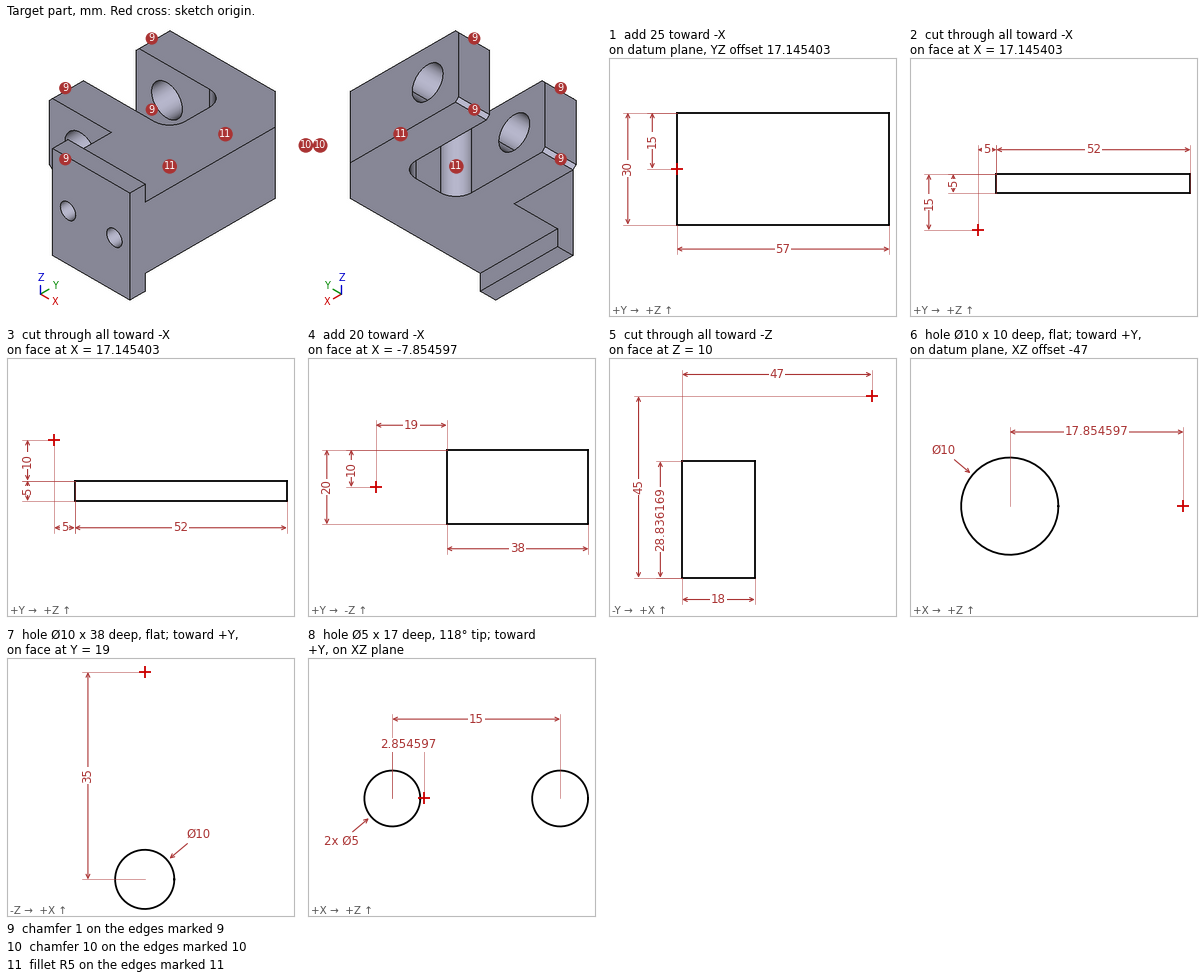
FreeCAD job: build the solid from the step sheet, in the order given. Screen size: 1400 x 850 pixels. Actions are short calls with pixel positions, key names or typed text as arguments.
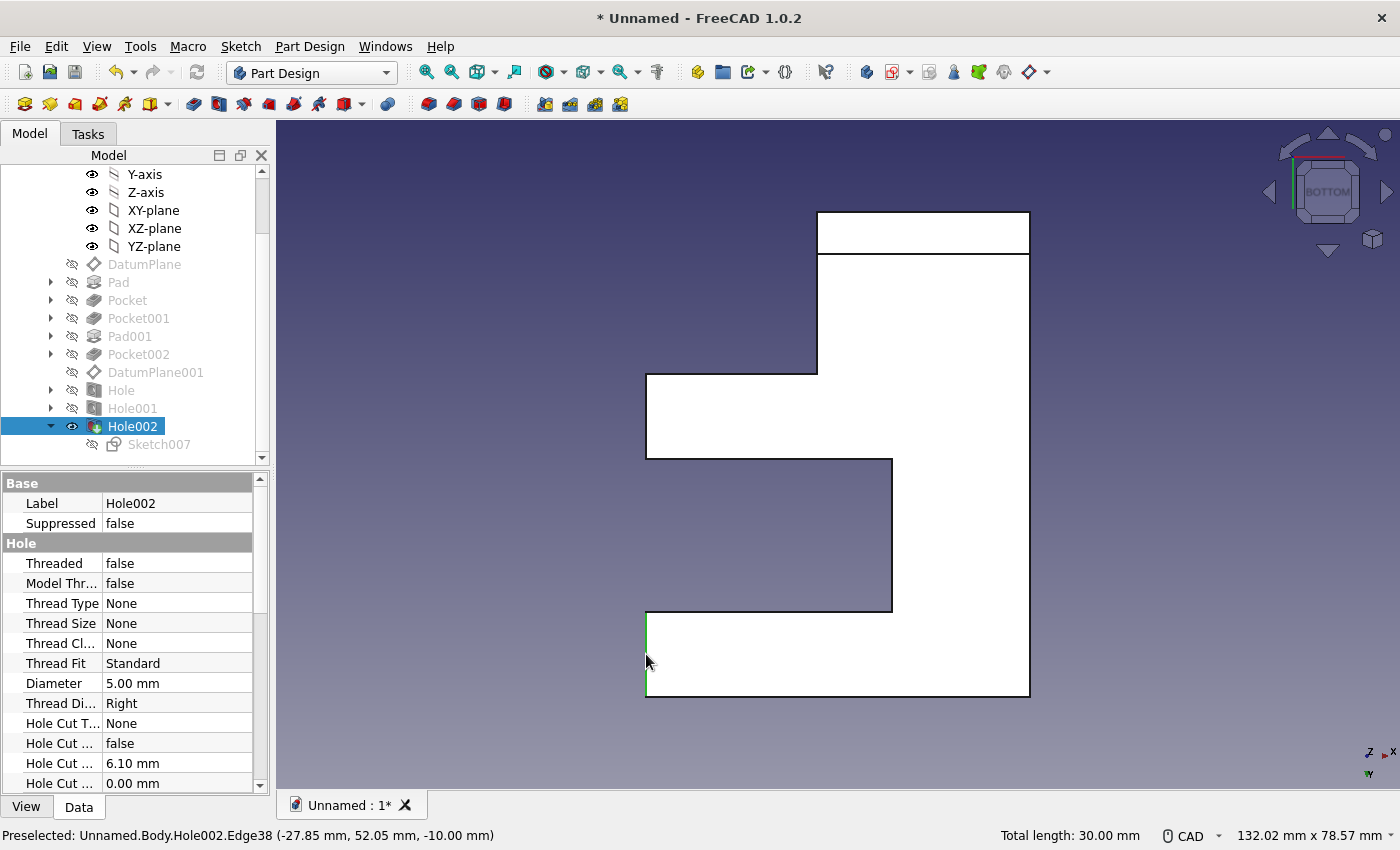
click(646, 415, ctrl)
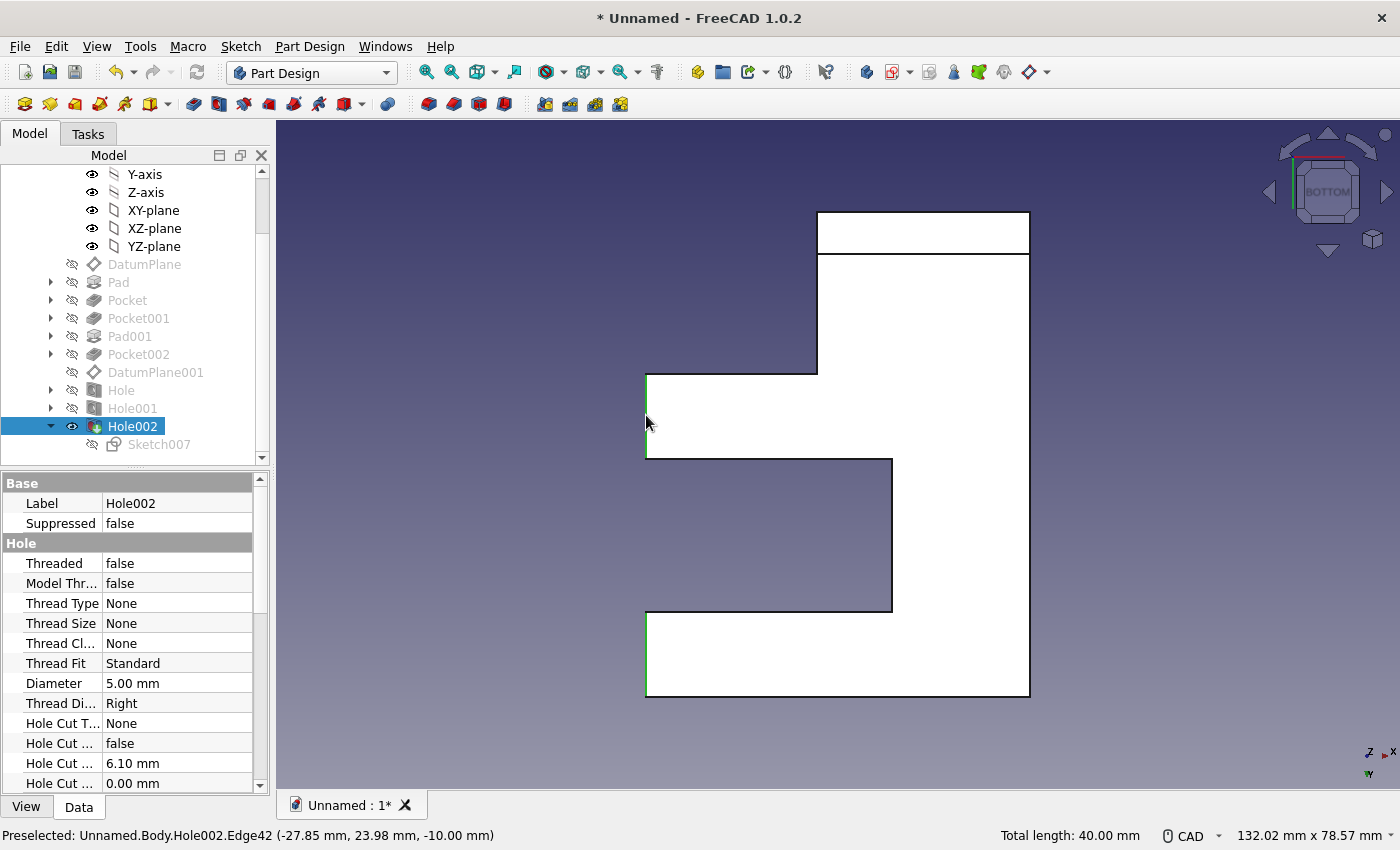
click(454, 104)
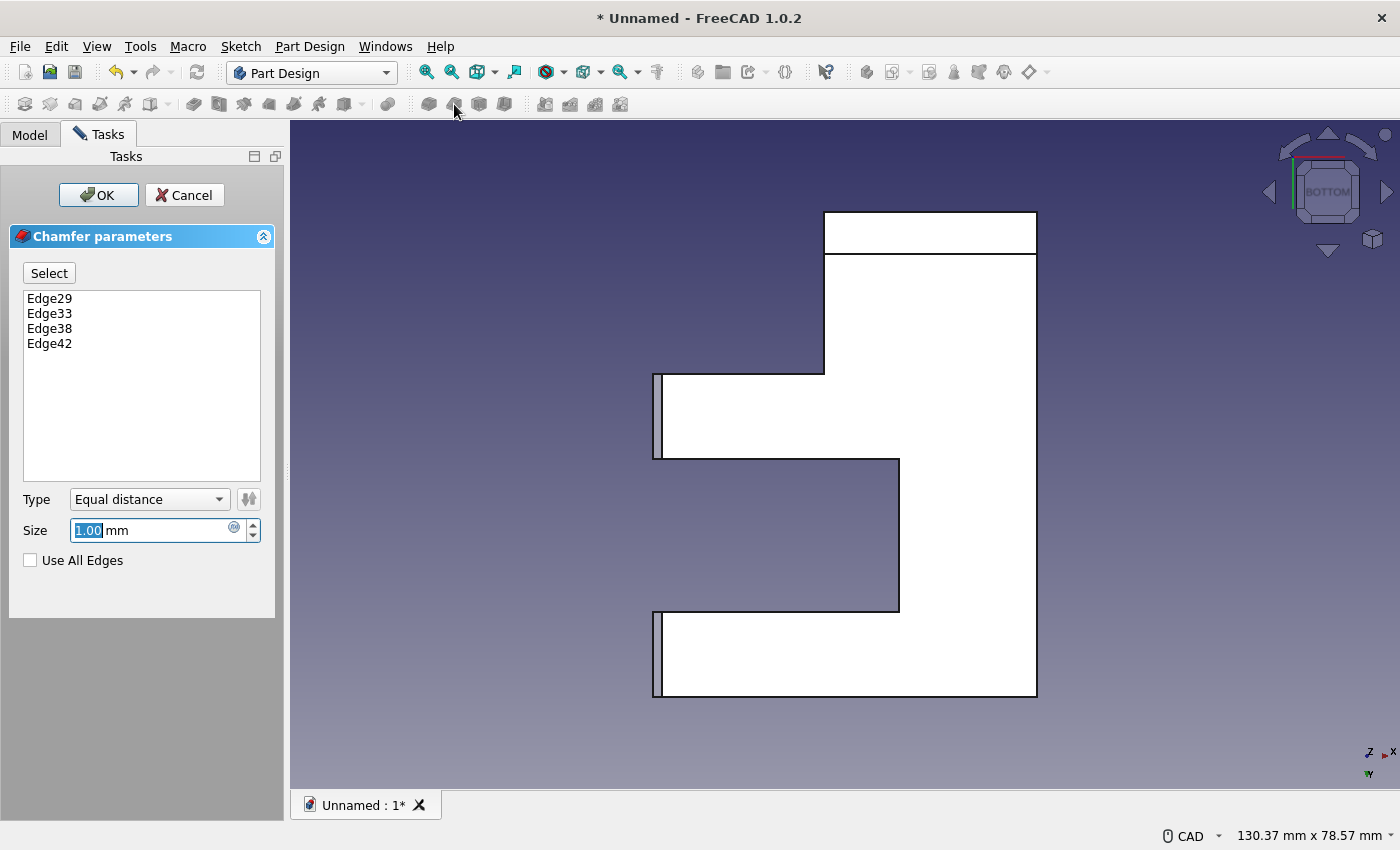
text(1)
key(Tab)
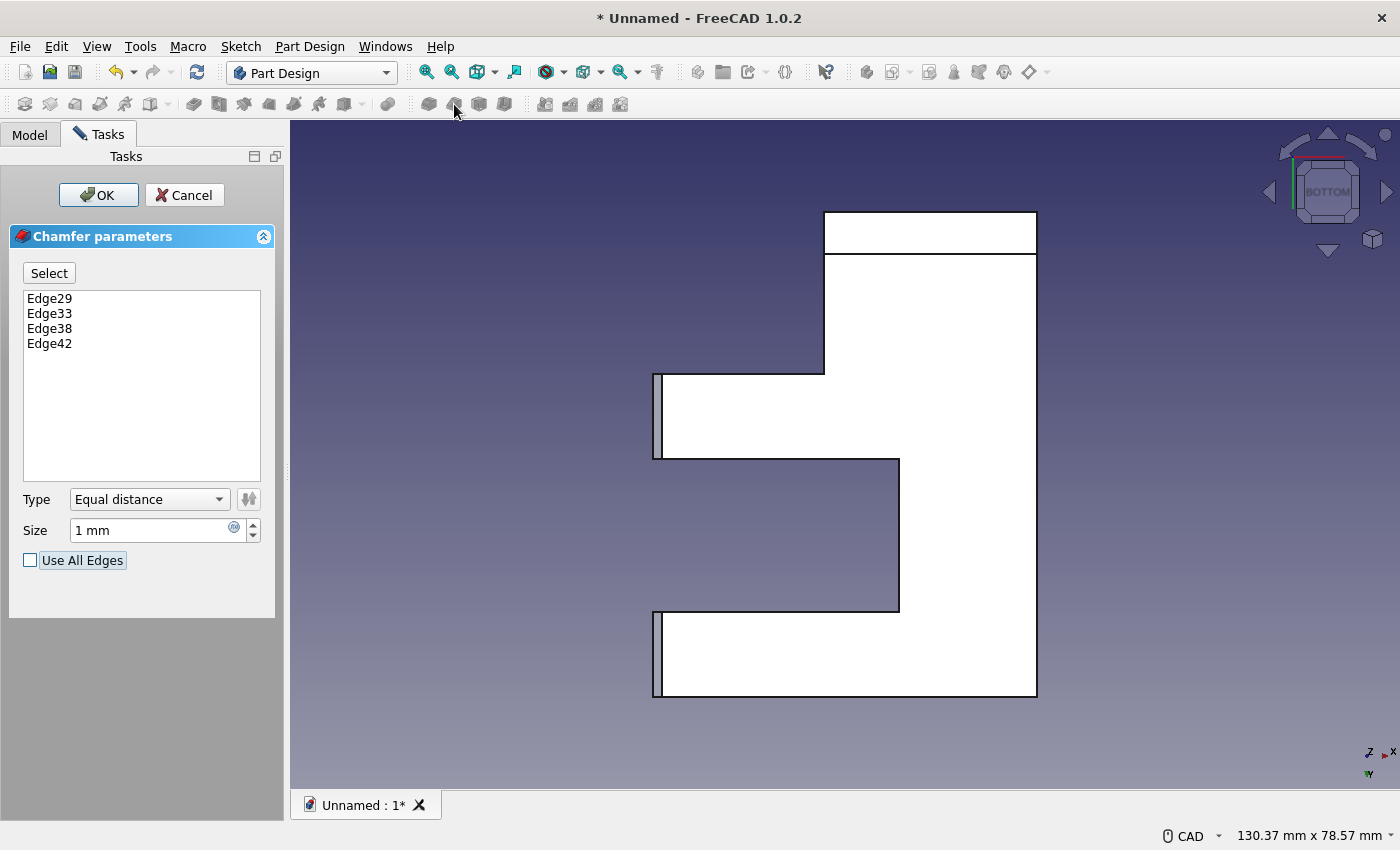
click(99, 195)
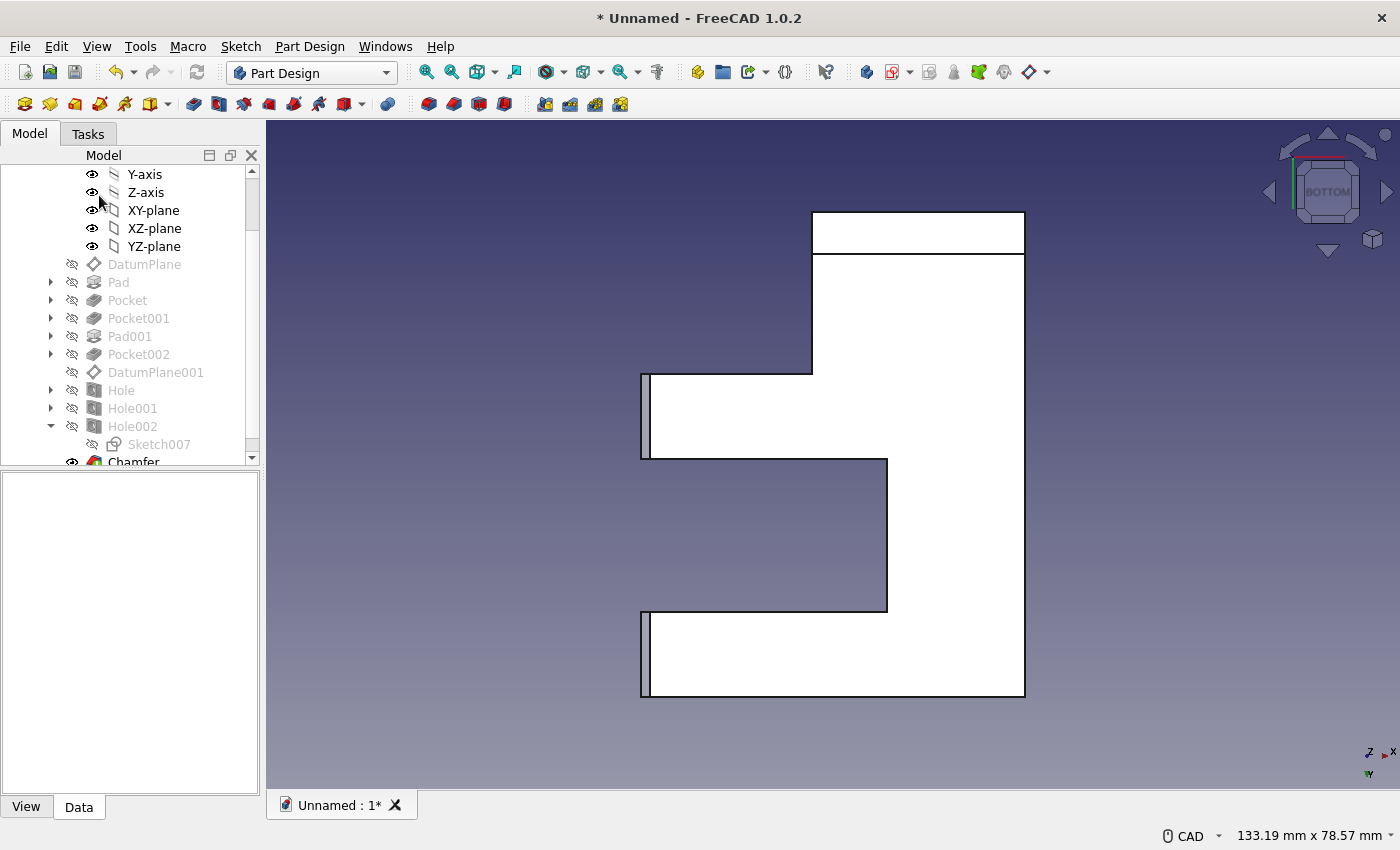
key(0)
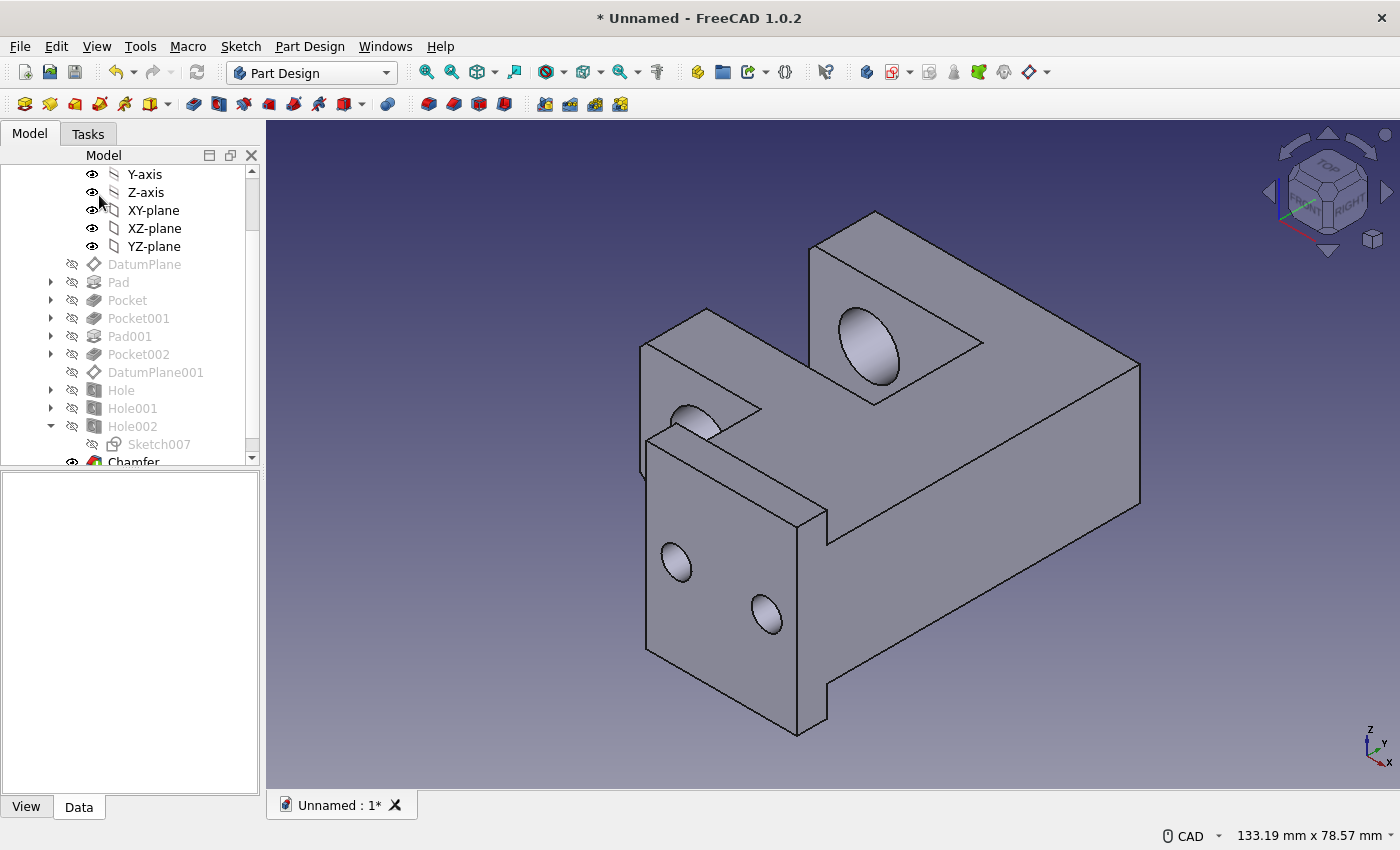
key(2)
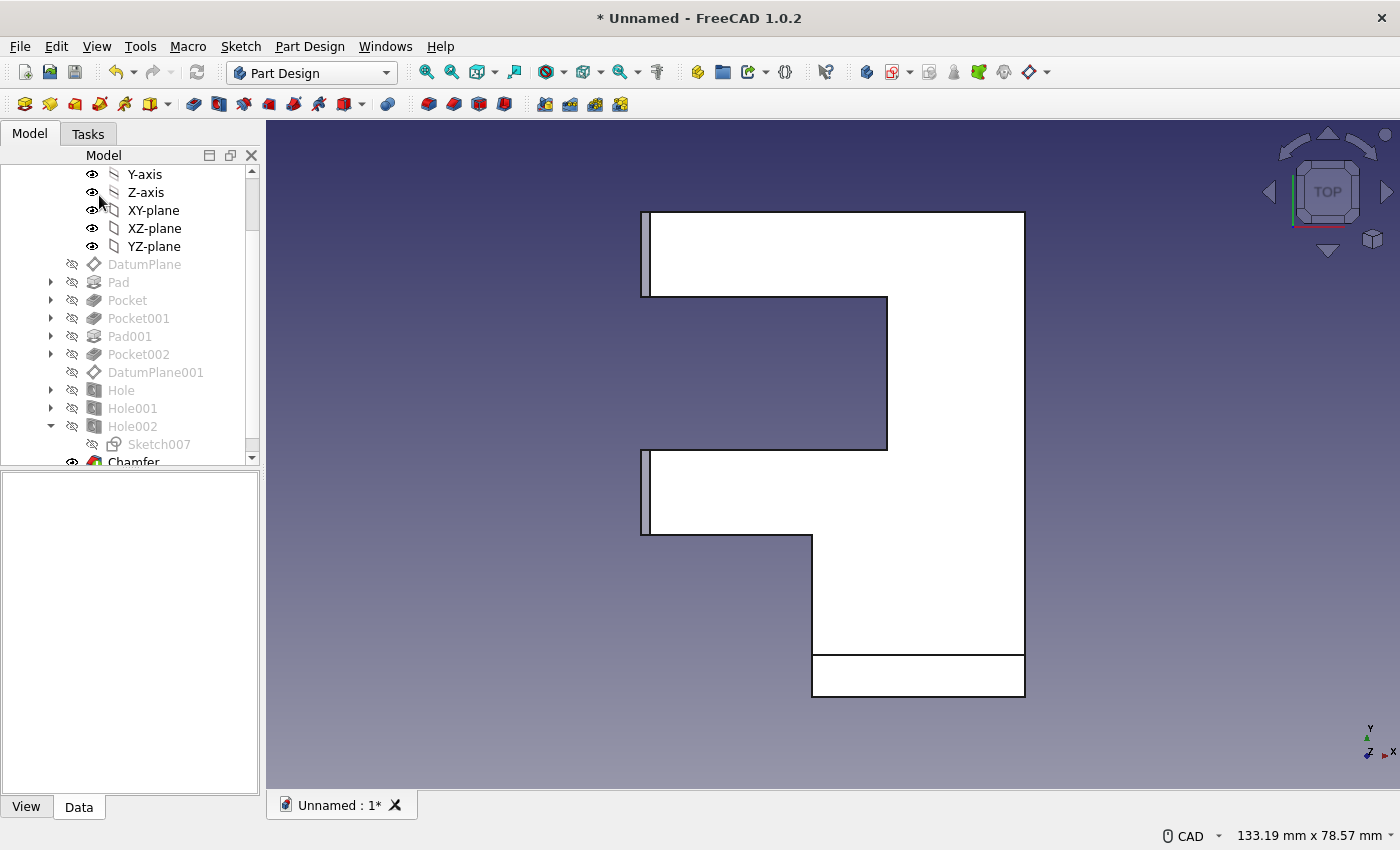
key(1)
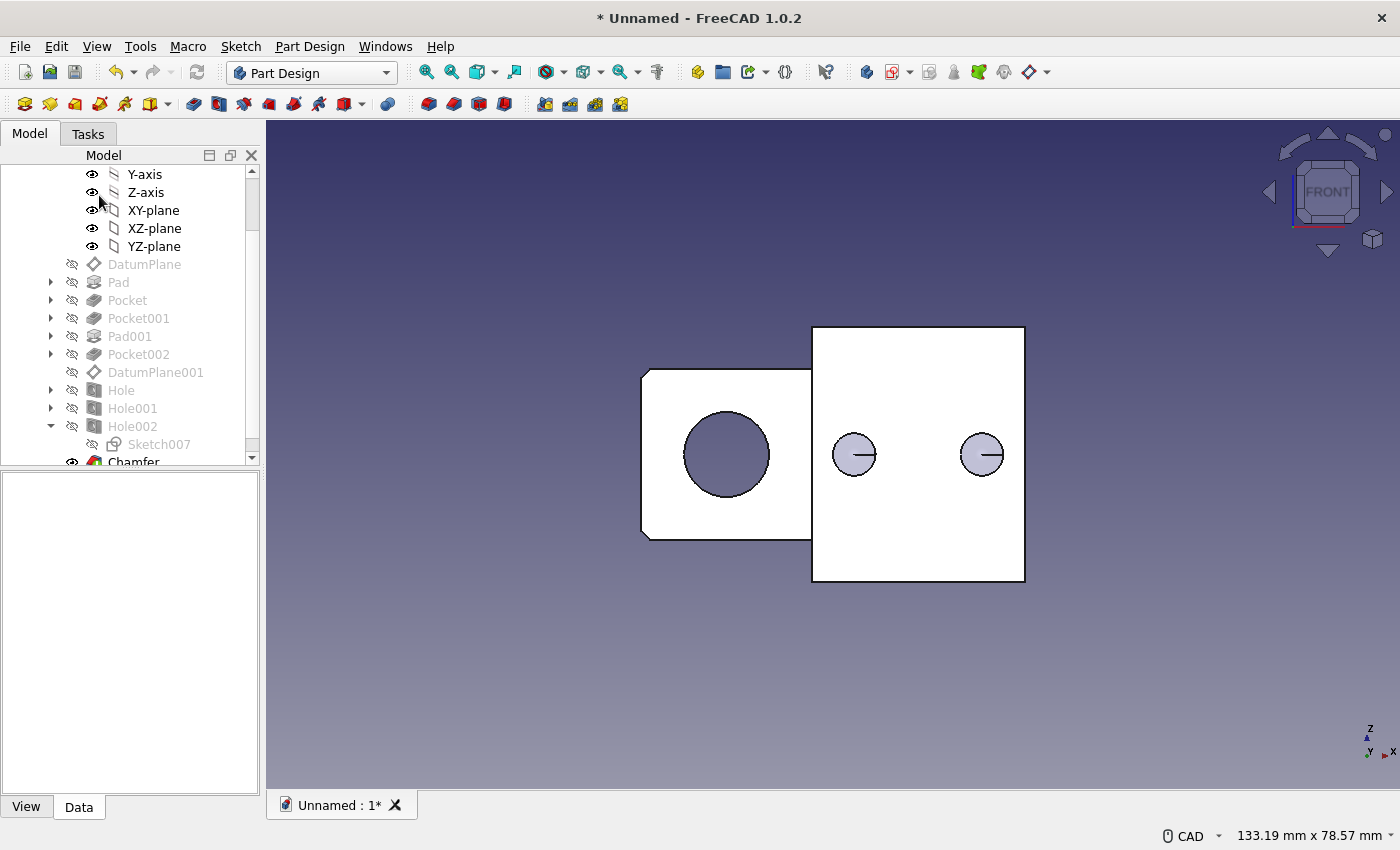
key(v)
key(f)